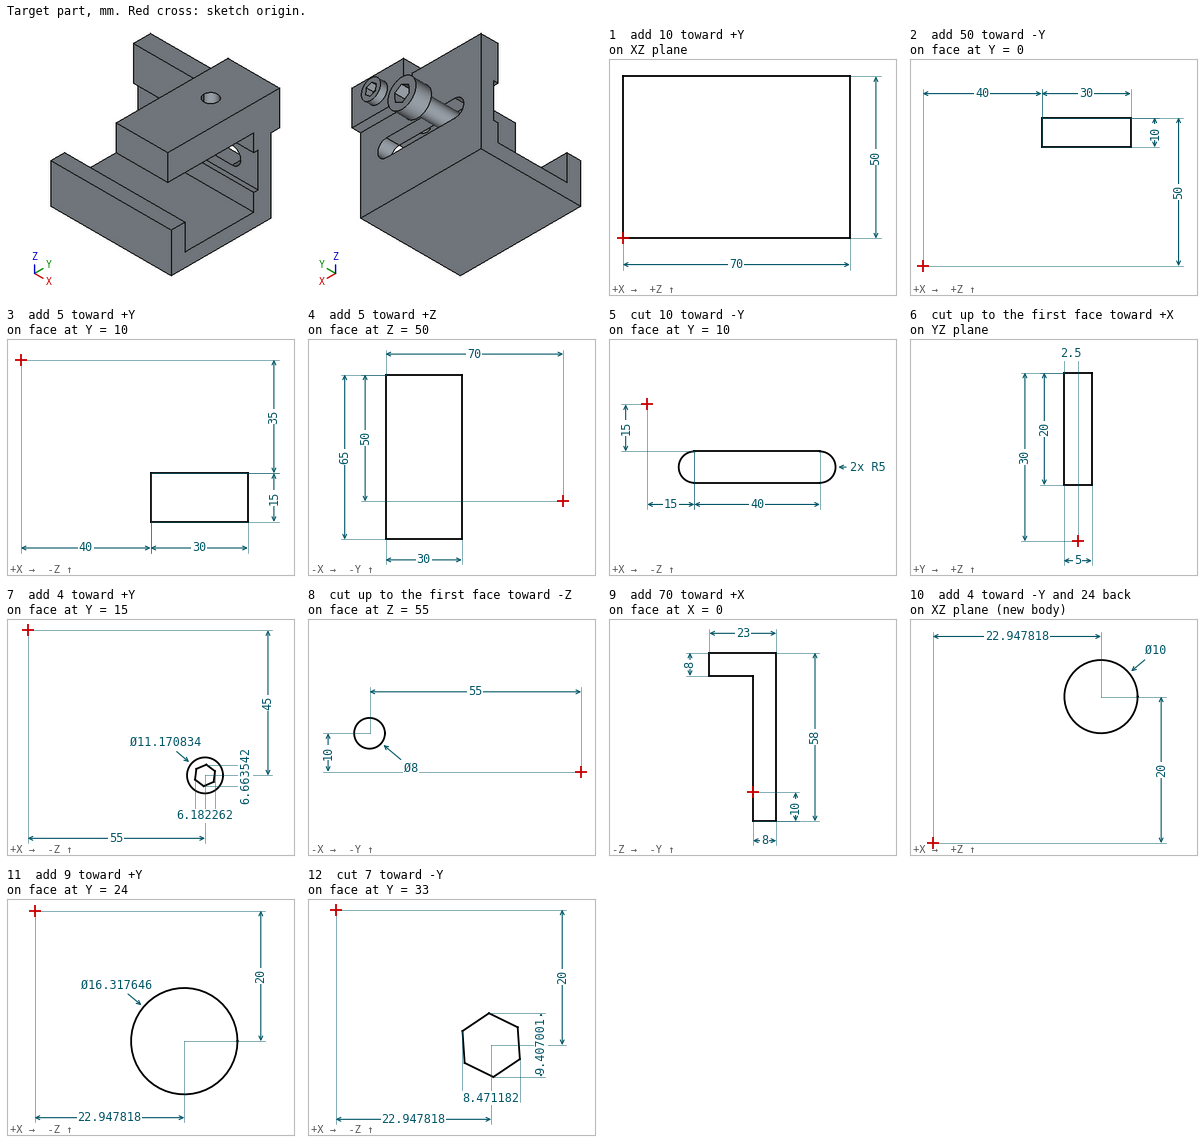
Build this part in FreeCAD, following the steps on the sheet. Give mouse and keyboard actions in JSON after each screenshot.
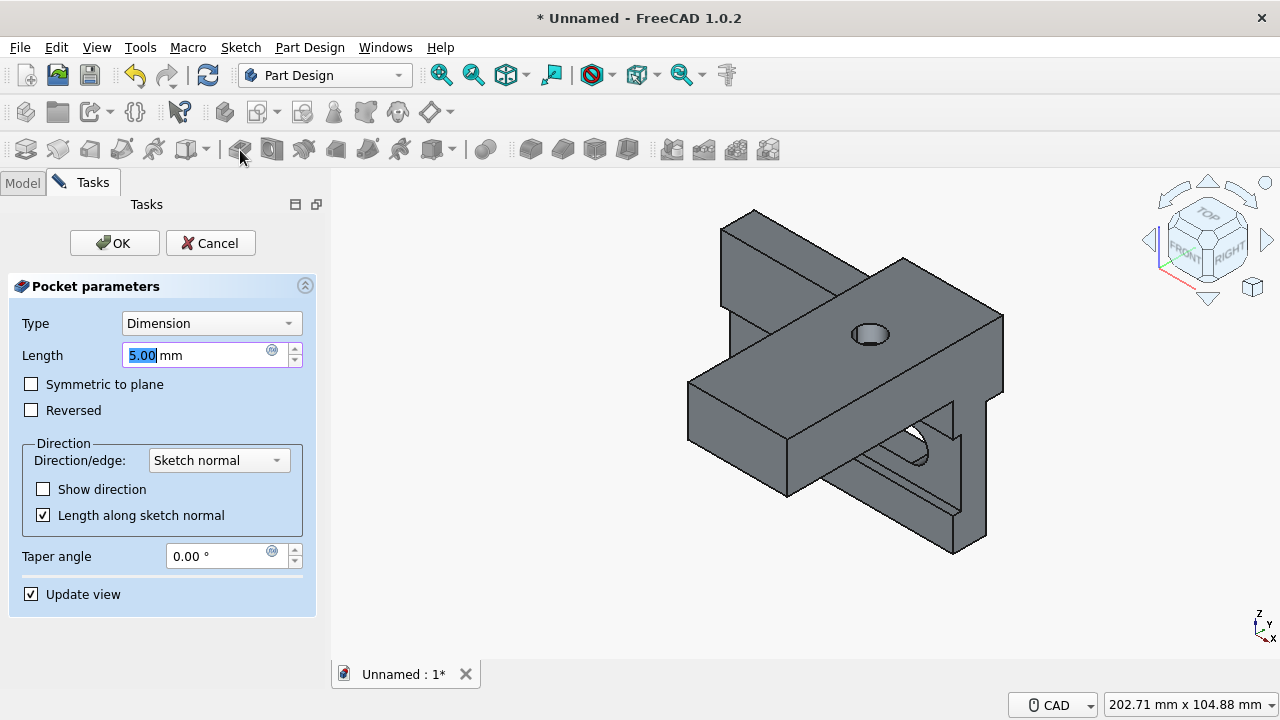
{"action": "left_click", "coordinate": [212, 324]}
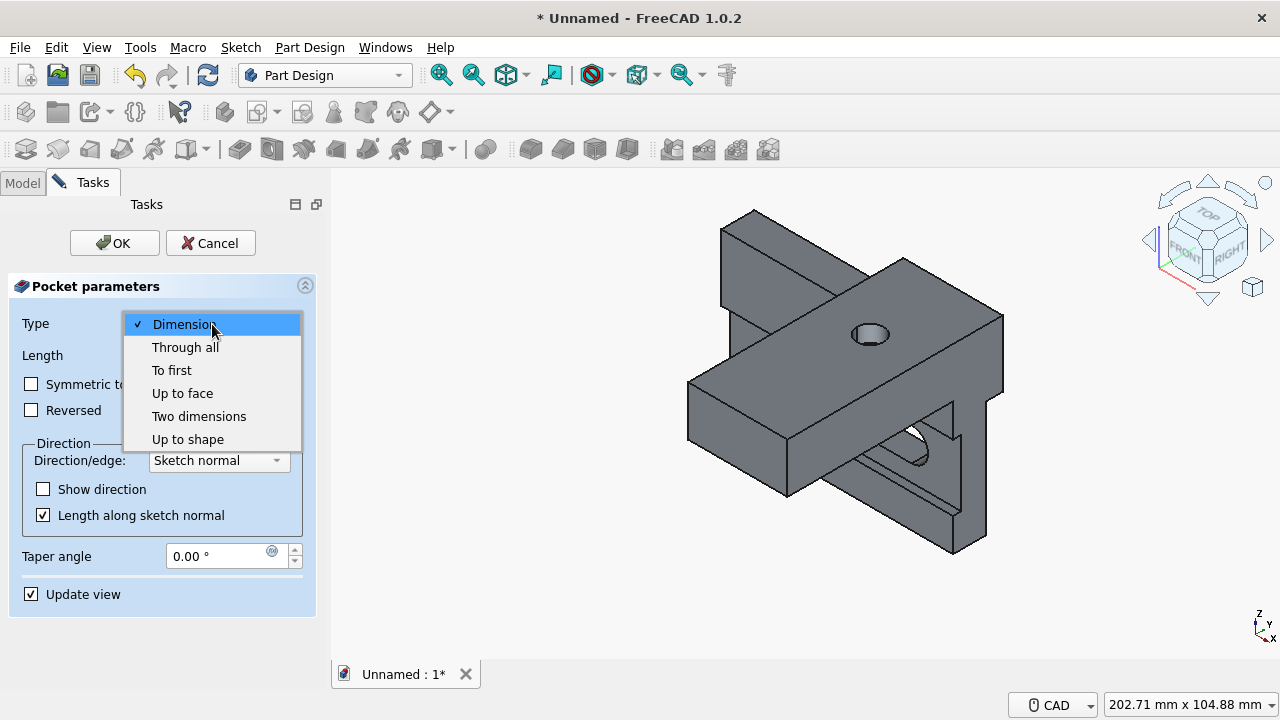
{"action": "left_click", "coordinate": [212, 370]}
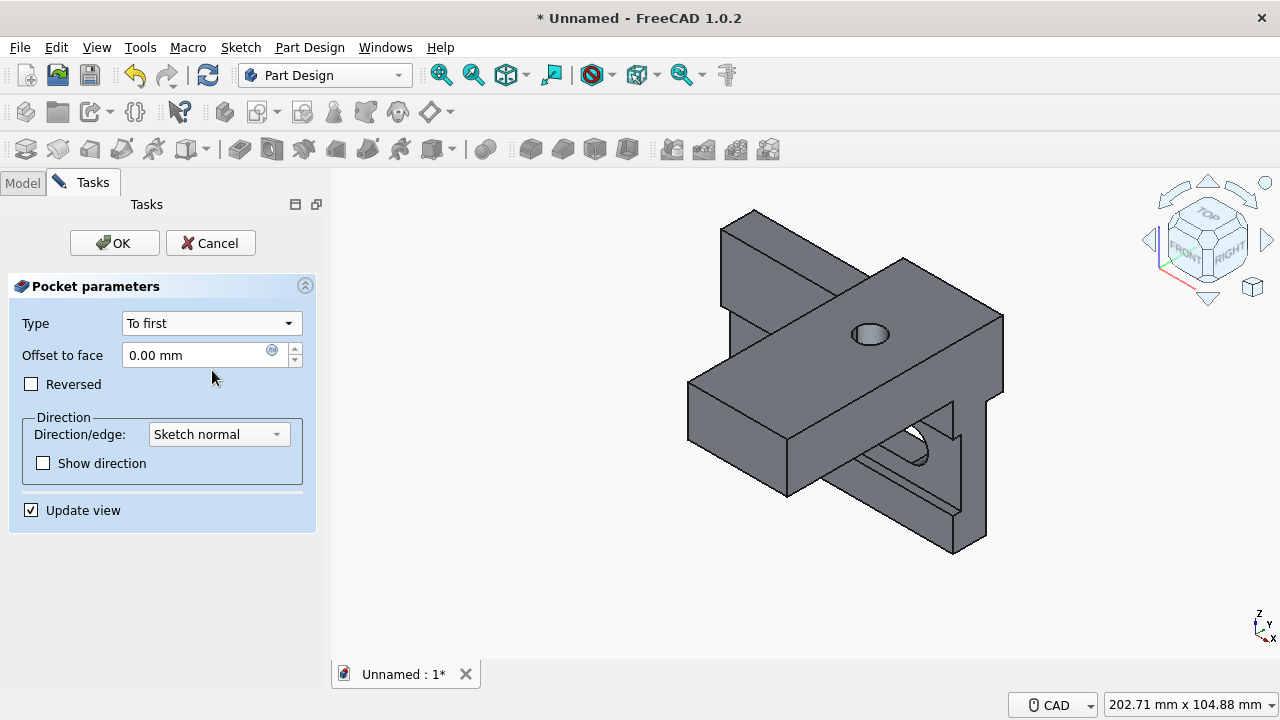
{"action": "left_click", "coordinate": [115, 243]}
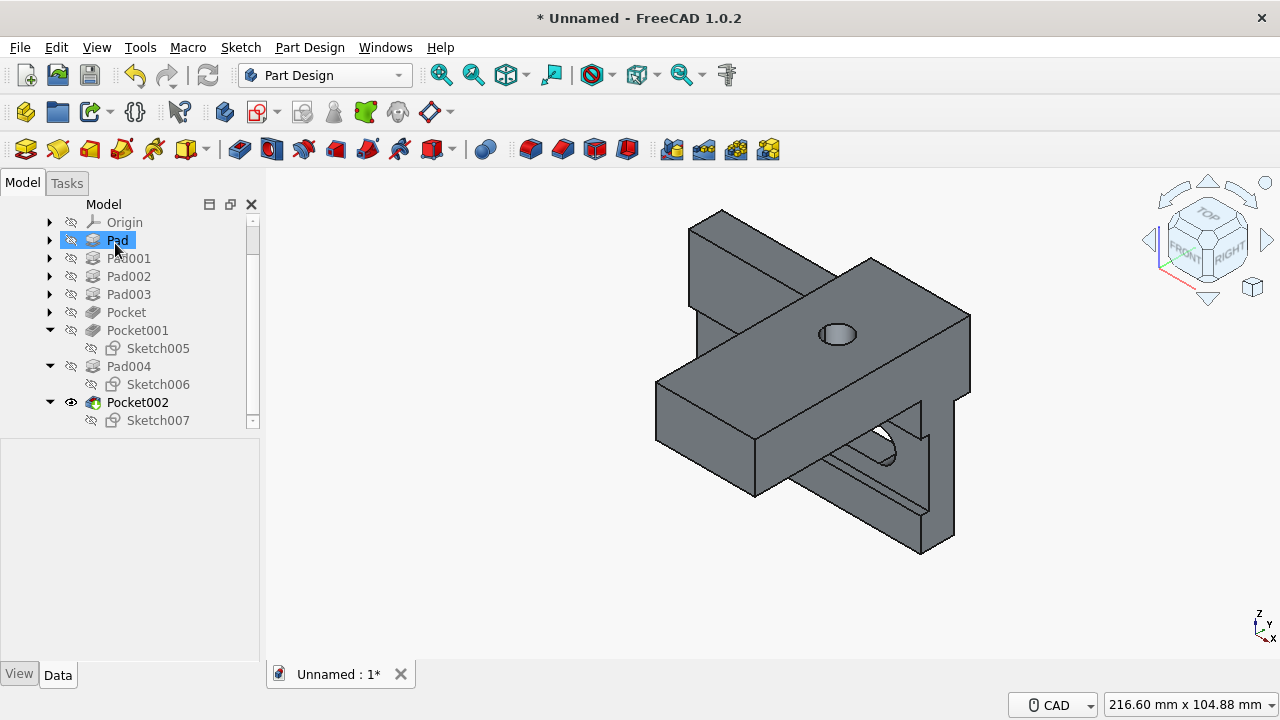
{"action": "key", "text": "6"}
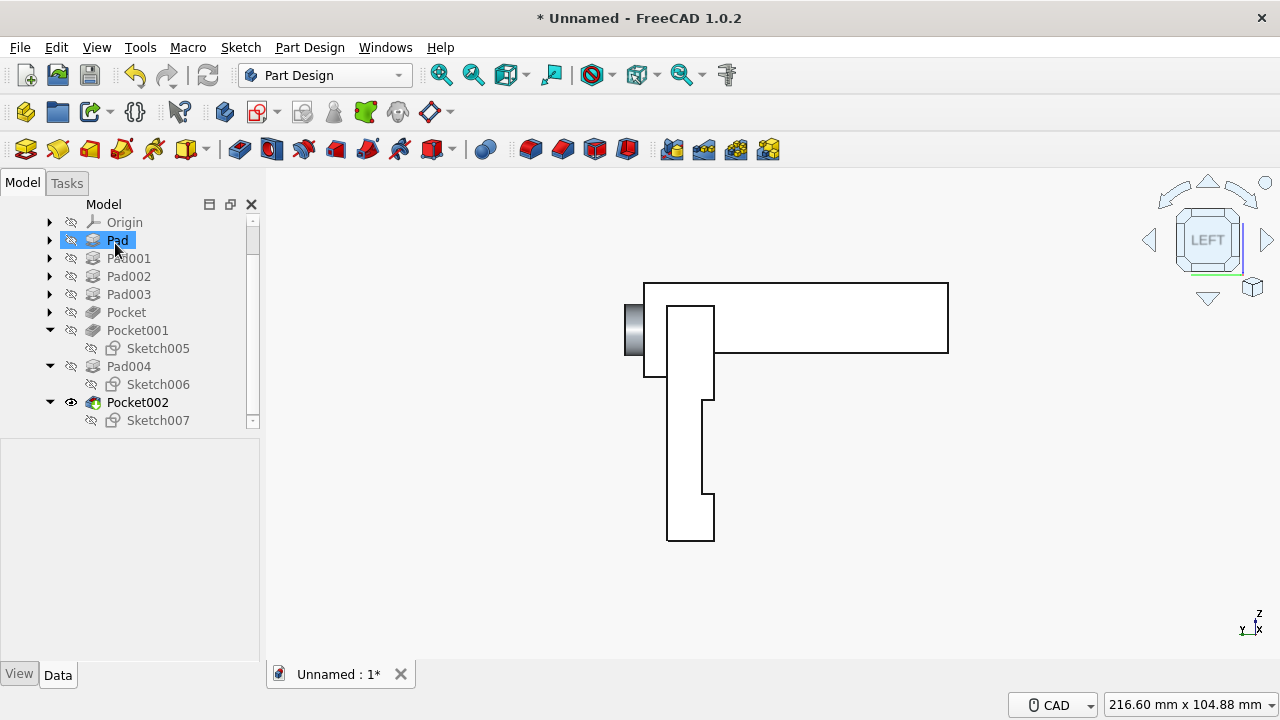
{"action": "left_click", "coordinate": [691, 356]}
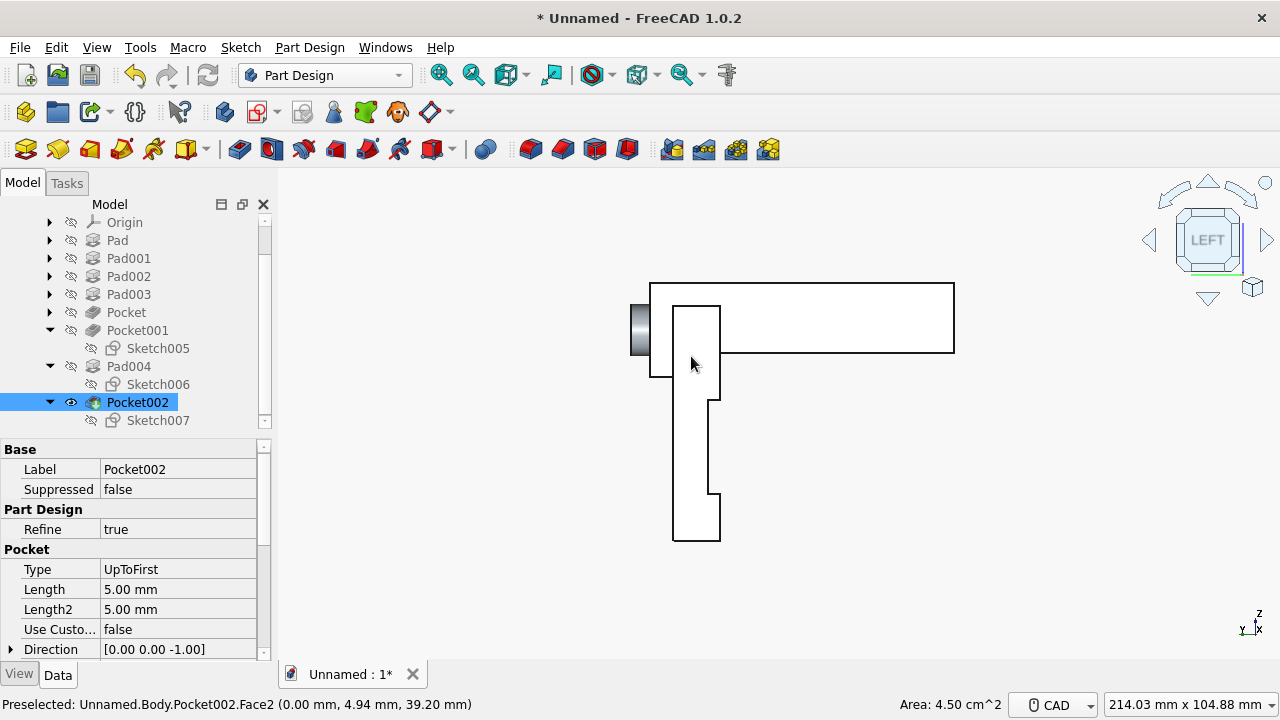
{"action": "left_click", "coordinate": [258, 112]}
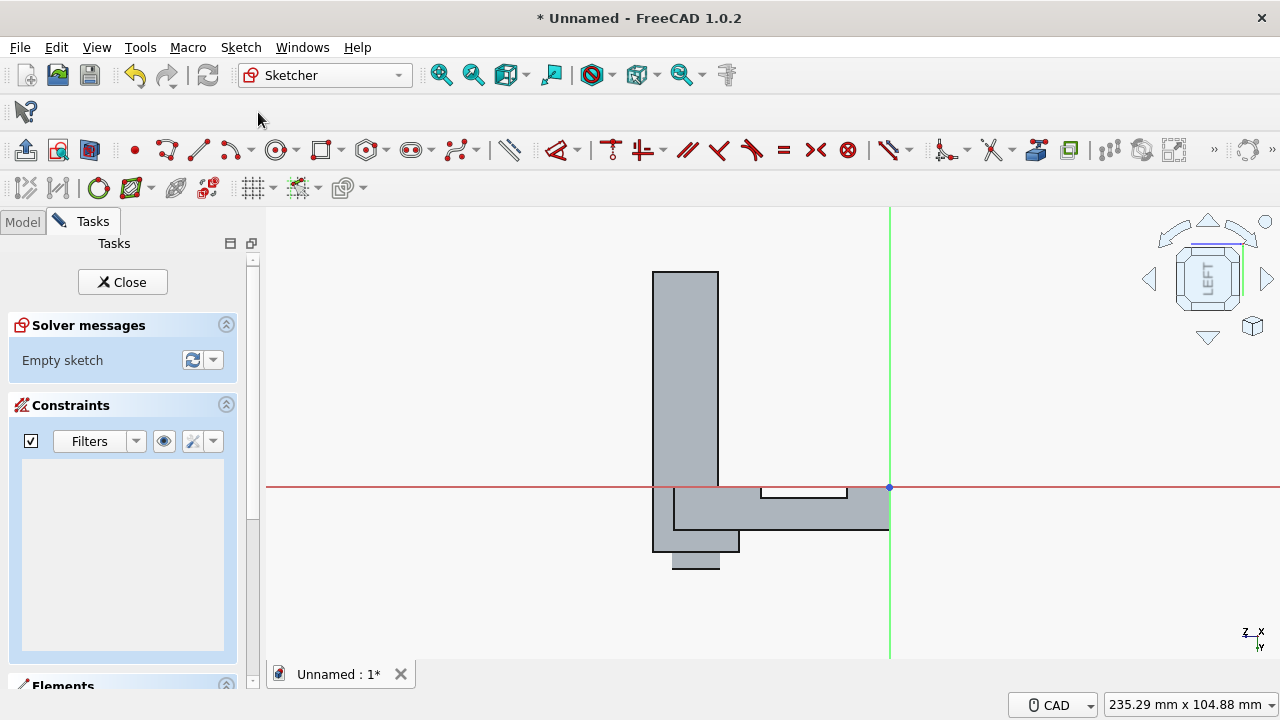
{"action": "left_click", "coordinate": [168, 150]}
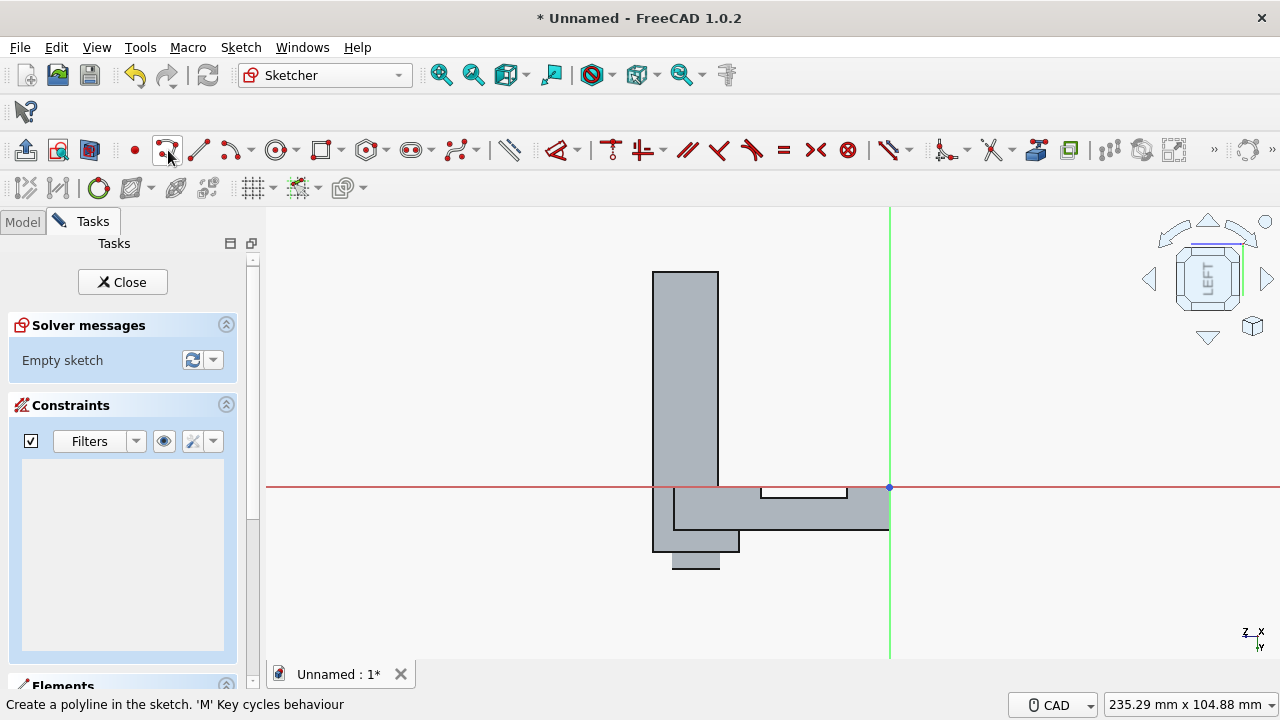
{"action": "left_click", "coordinate": [890, 530]}
{"action": "left_click", "coordinate": [924, 530]}
{"action": "left_click", "coordinate": [924, 280]}
{"action": "left_click", "coordinate": [825, 280]}
{"action": "left_click", "coordinate": [825, 315]}
{"action": "left_click", "coordinate": [881, 315]}
{"action": "left_click", "coordinate": [890, 531]}
{"action": "key", "text": "Escape"}
{"action": "key", "text": "Escape"}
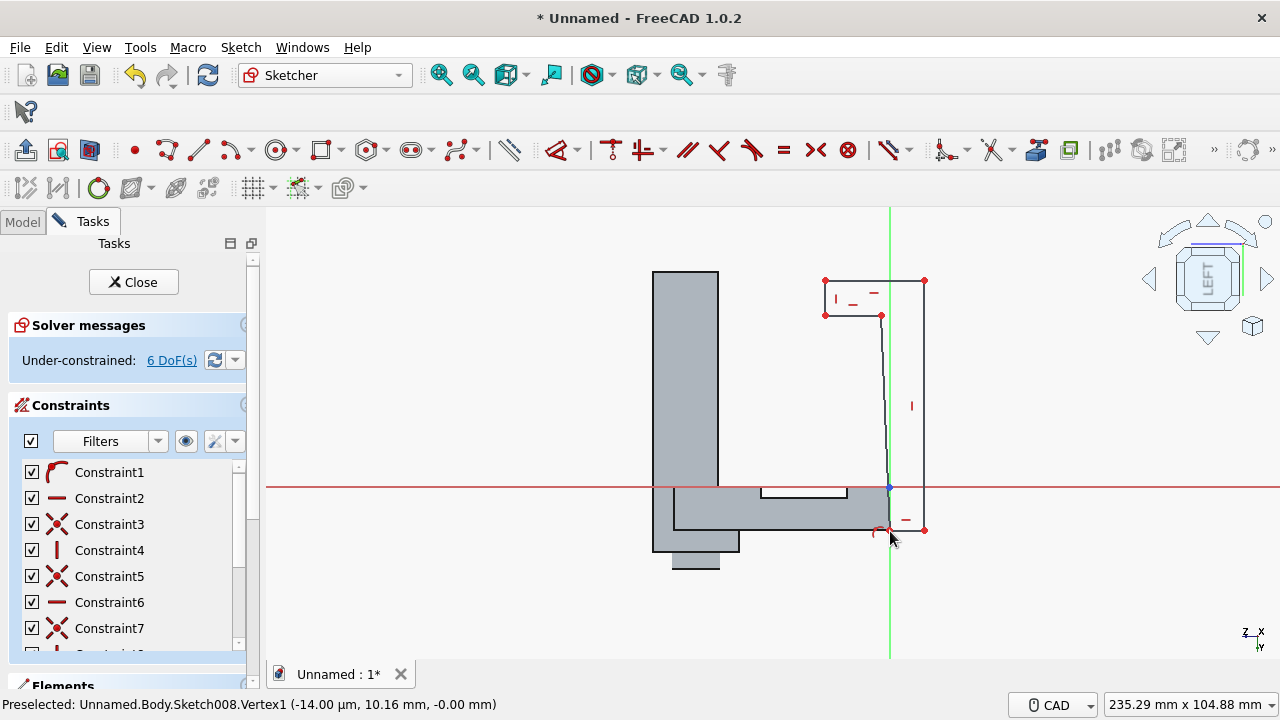
{"action": "left_click", "coordinate": [887, 467]}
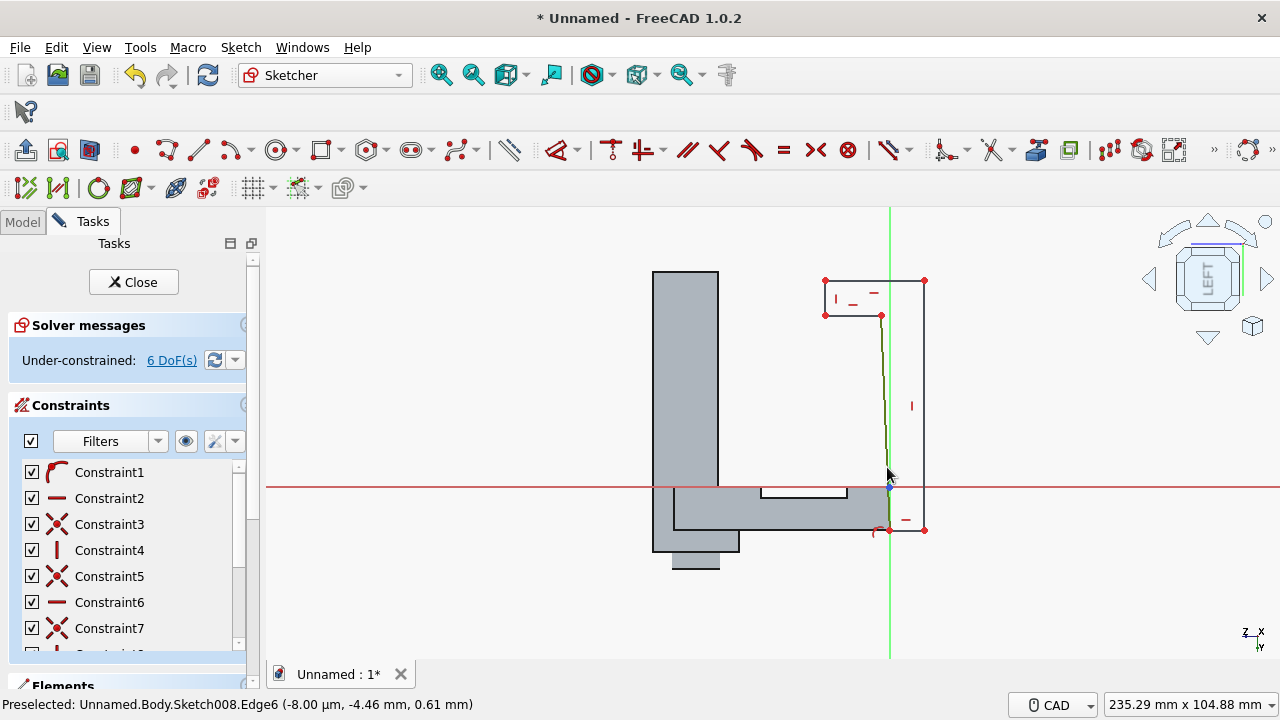
{"action": "key", "text": "v"}